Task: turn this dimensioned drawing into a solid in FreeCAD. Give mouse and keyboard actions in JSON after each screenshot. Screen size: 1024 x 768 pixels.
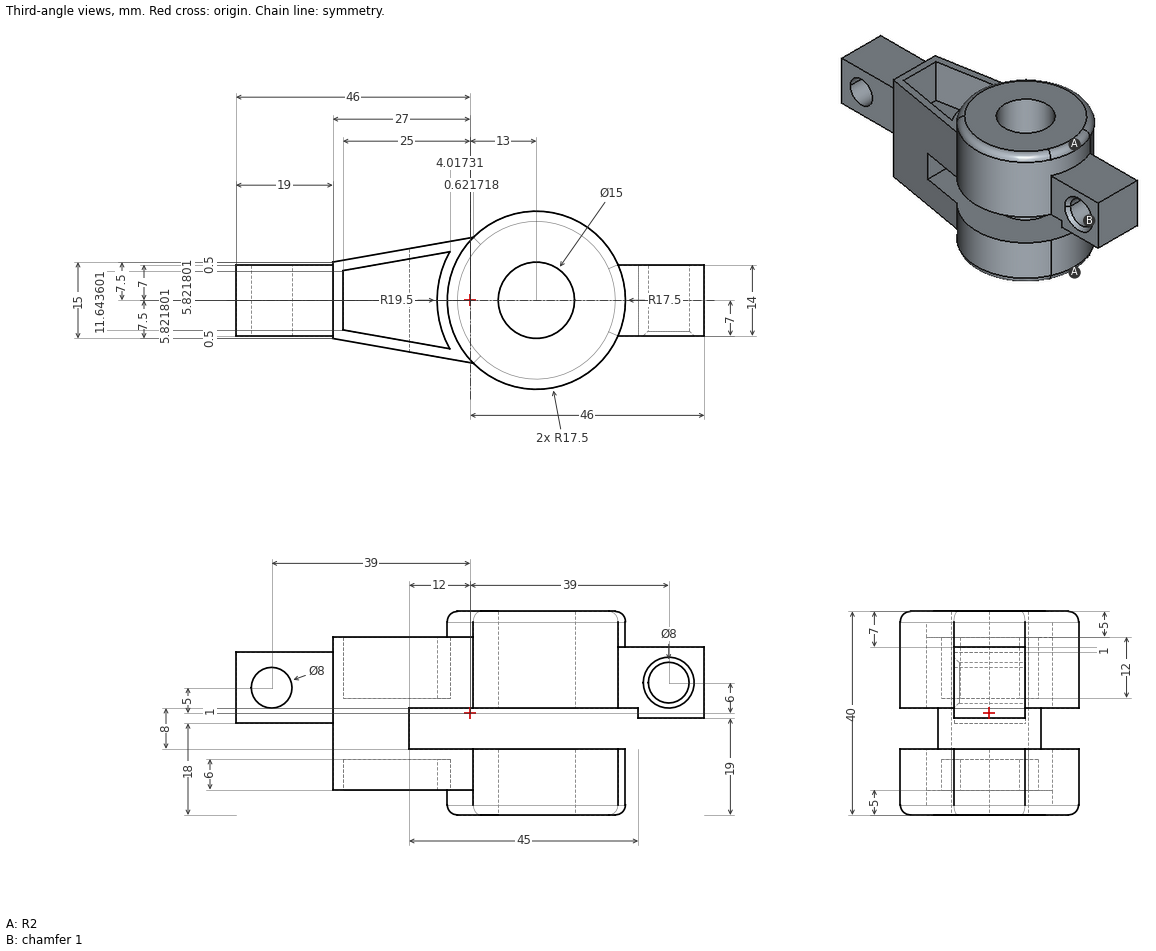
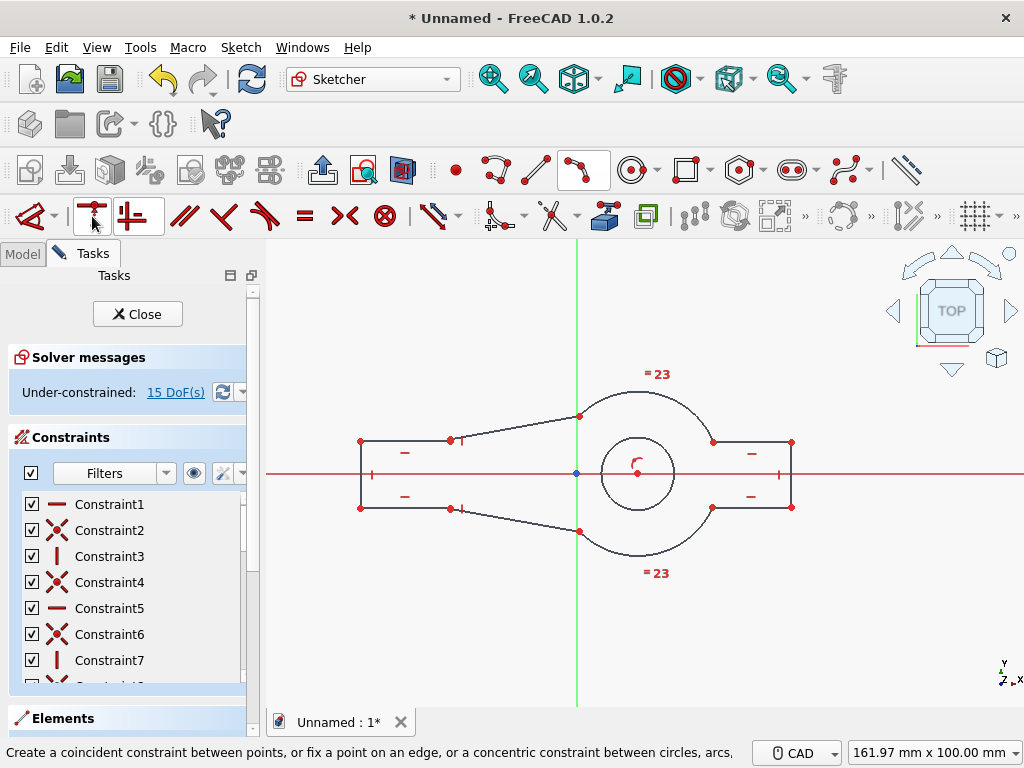
{"action": "left_click", "coordinate": [791, 442]}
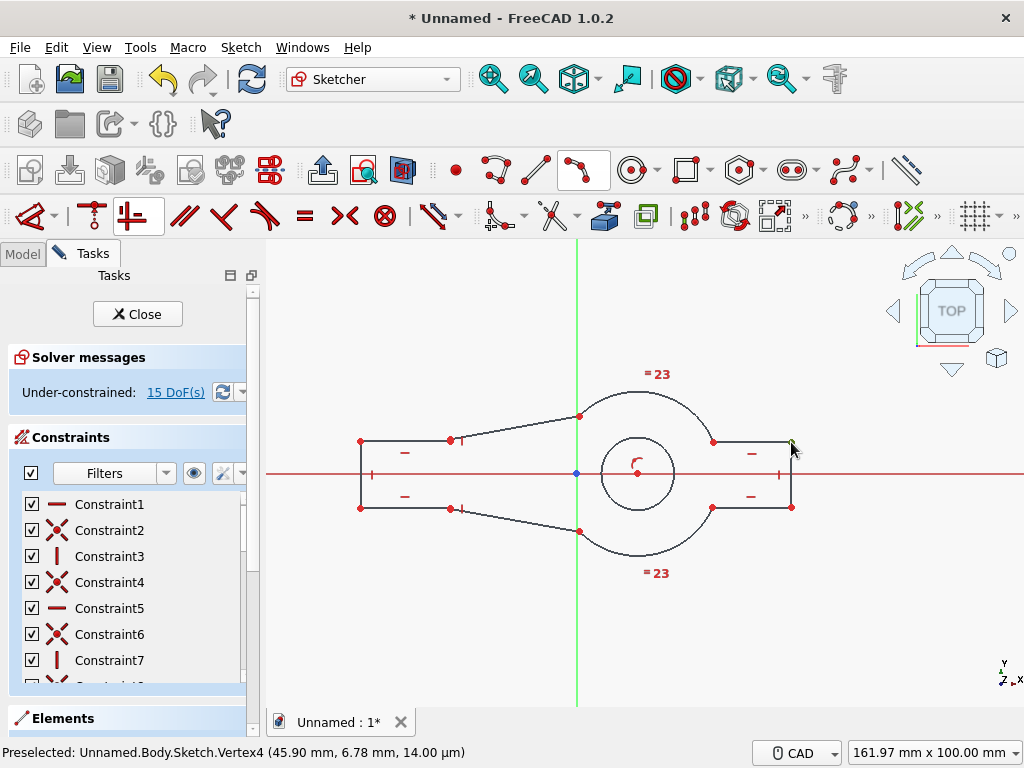
{"action": "left_click", "coordinate": [361, 441]}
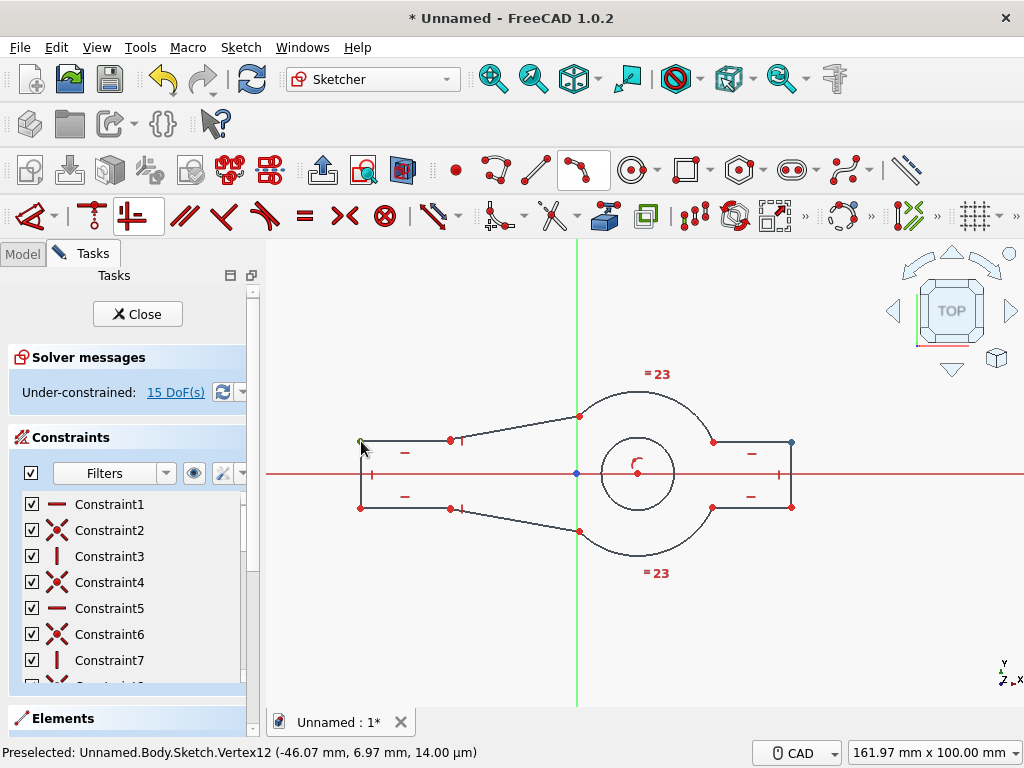
{"action": "left_click", "coordinate": [577, 650]}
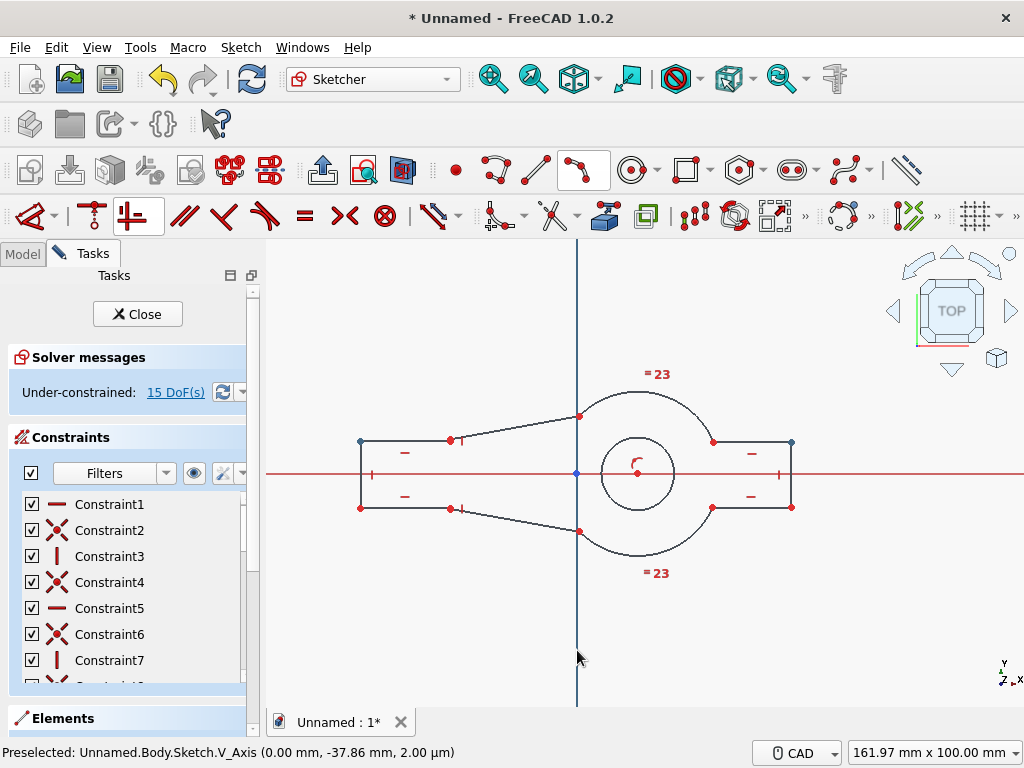
{"action": "left_click", "coordinate": [346, 216]}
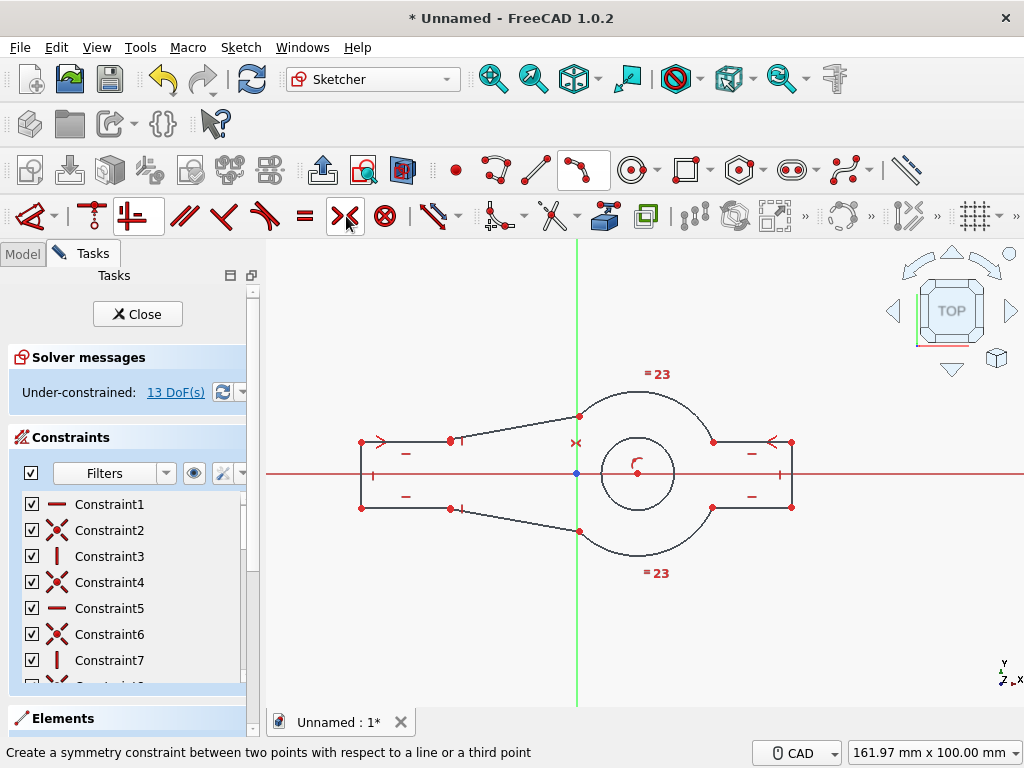
{"action": "scroll", "coordinate": [451, 442], "scroll_direction": "up", "scroll_amount": 8}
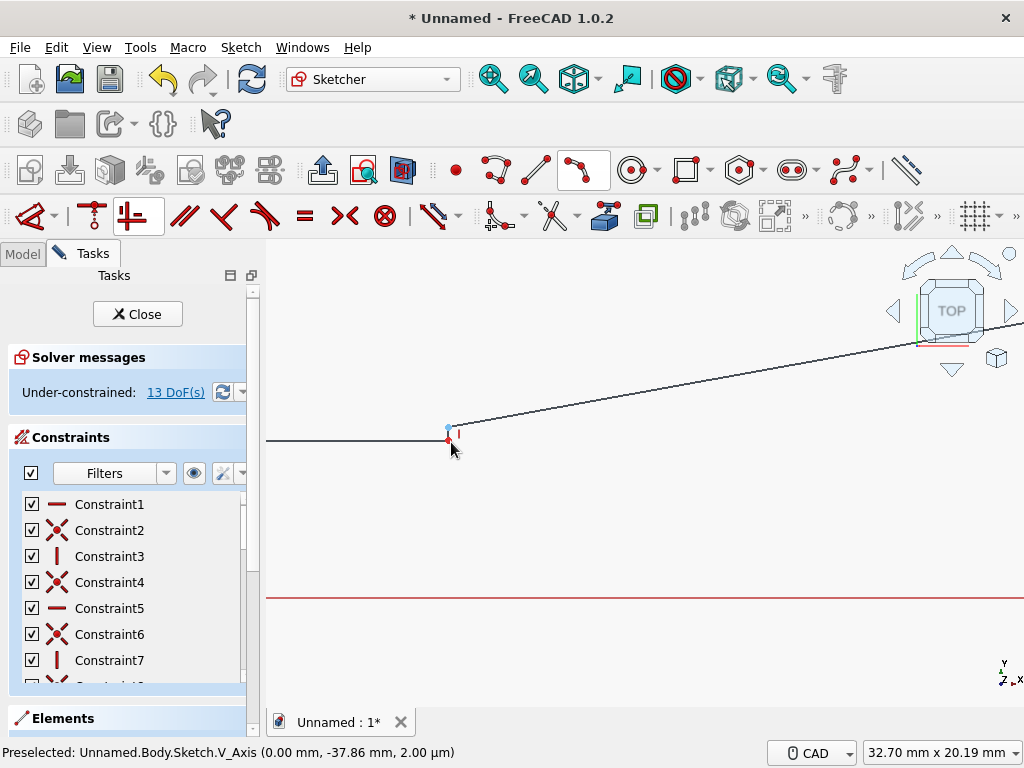
{"action": "left_click", "coordinate": [448, 441]}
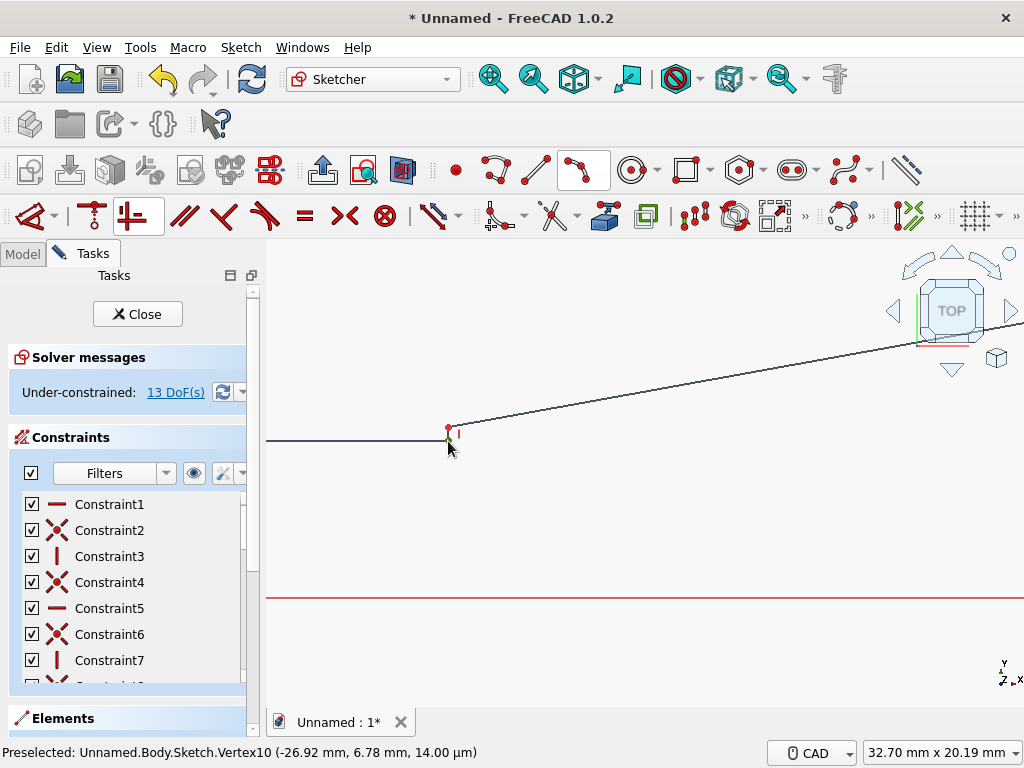
{"action": "scroll", "coordinate": [451, 441], "scroll_direction": "down", "scroll_amount": 8}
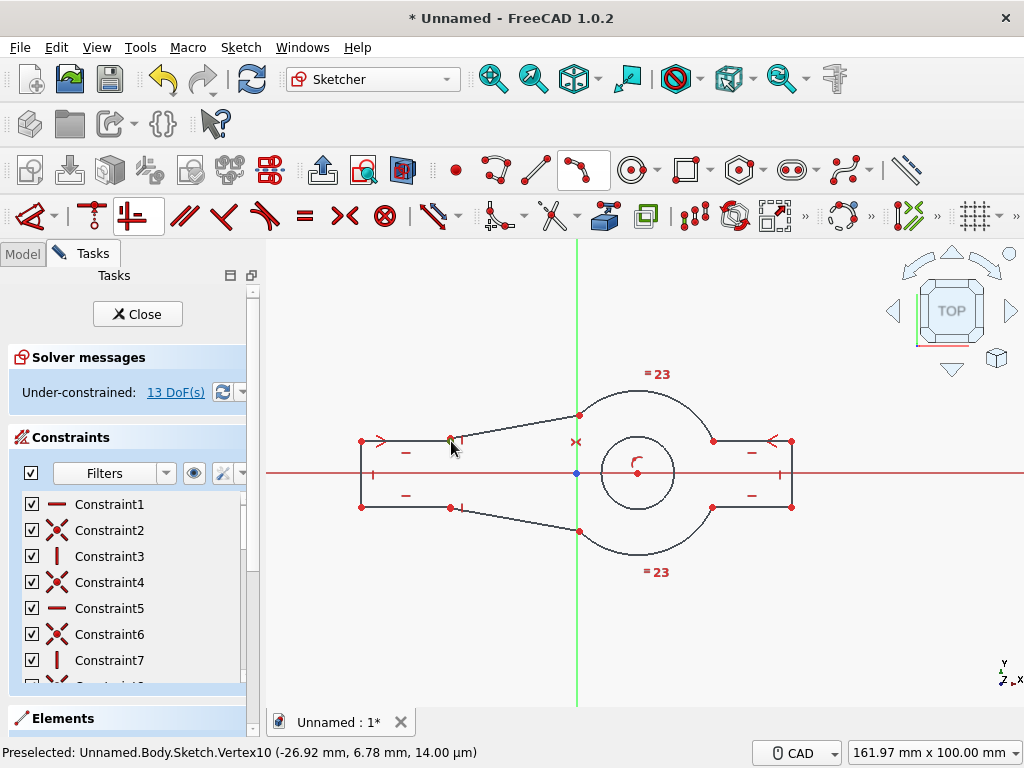
{"action": "scroll", "coordinate": [451, 507], "scroll_direction": "up", "scroll_amount": 13}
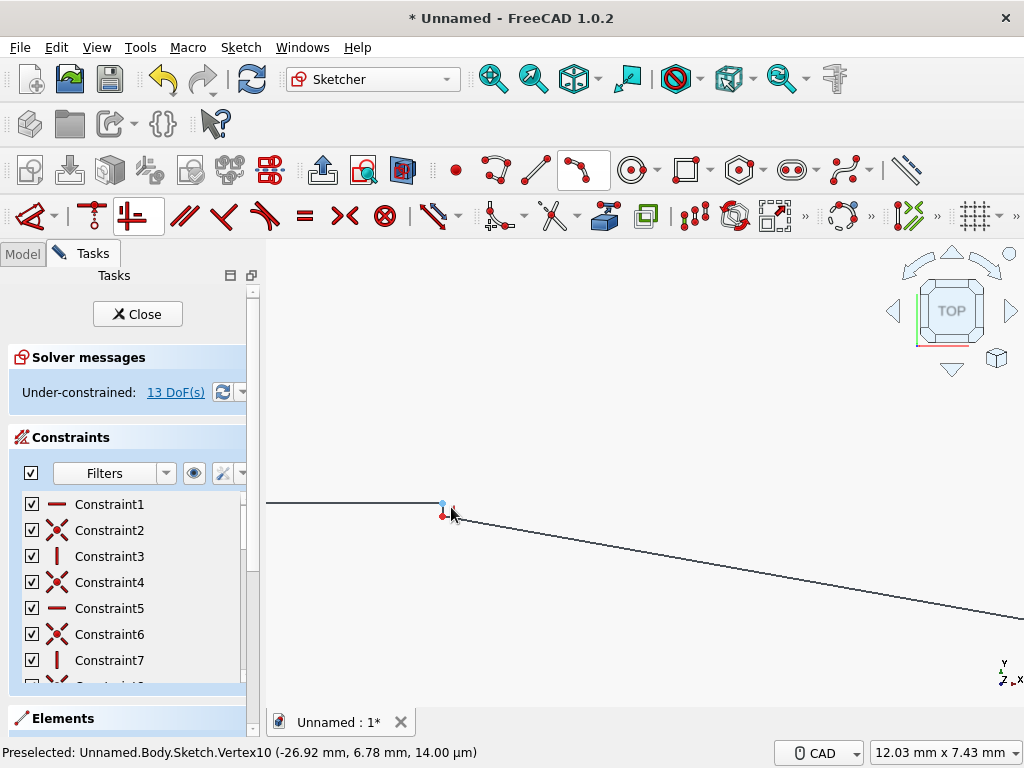
{"action": "left_click", "coordinate": [443, 503]}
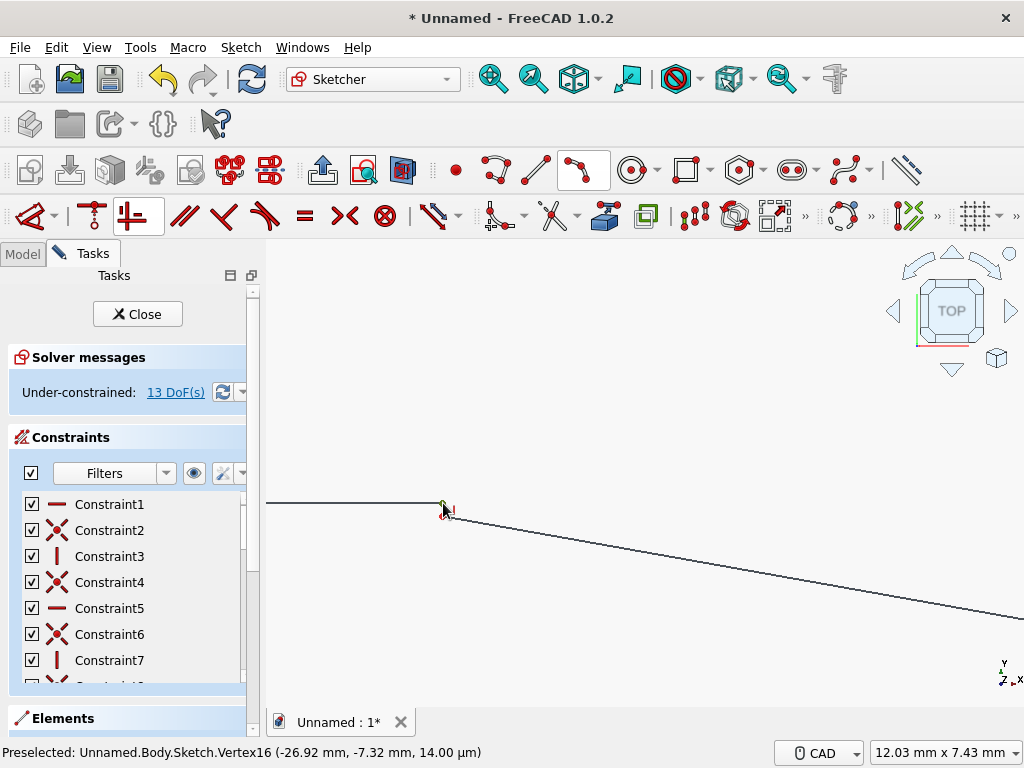
{"action": "scroll", "coordinate": [451, 508], "scroll_direction": "down", "scroll_amount": 13}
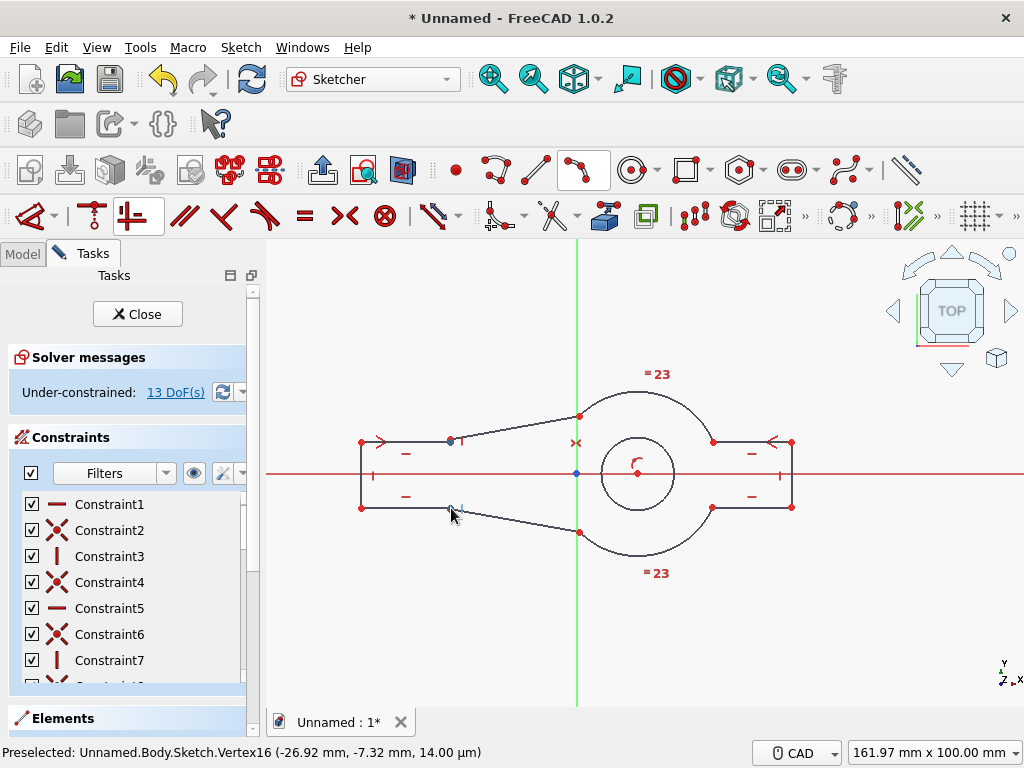
{"action": "left_click", "coordinate": [415, 474]}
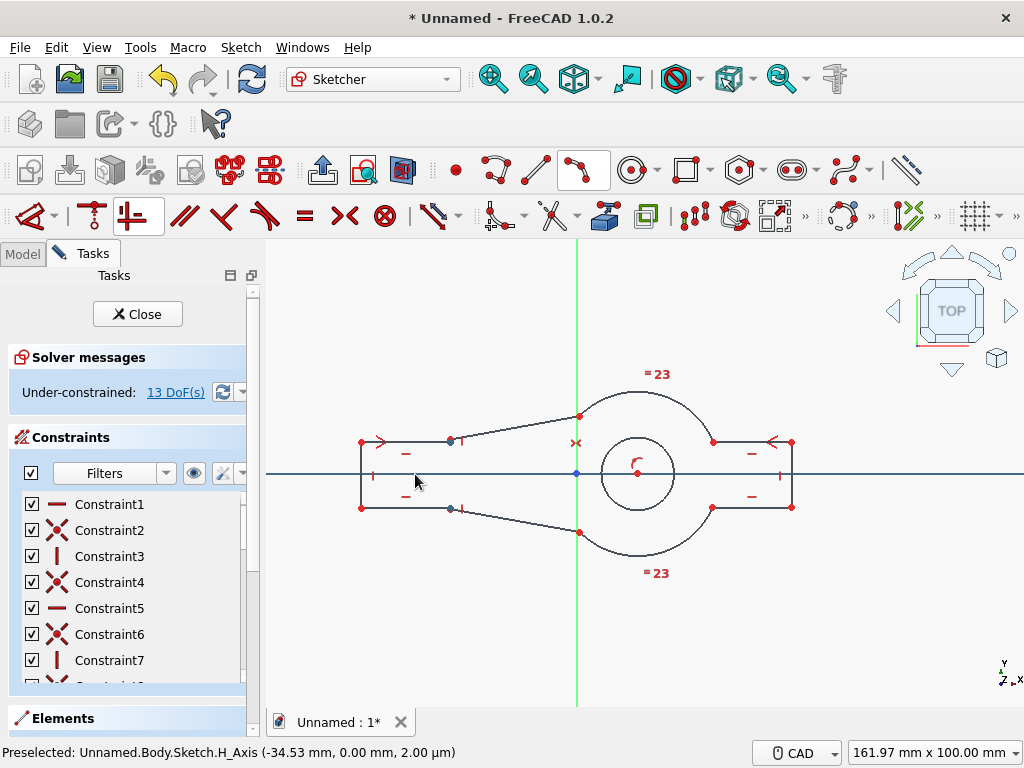
{"action": "left_click", "coordinate": [346, 216]}